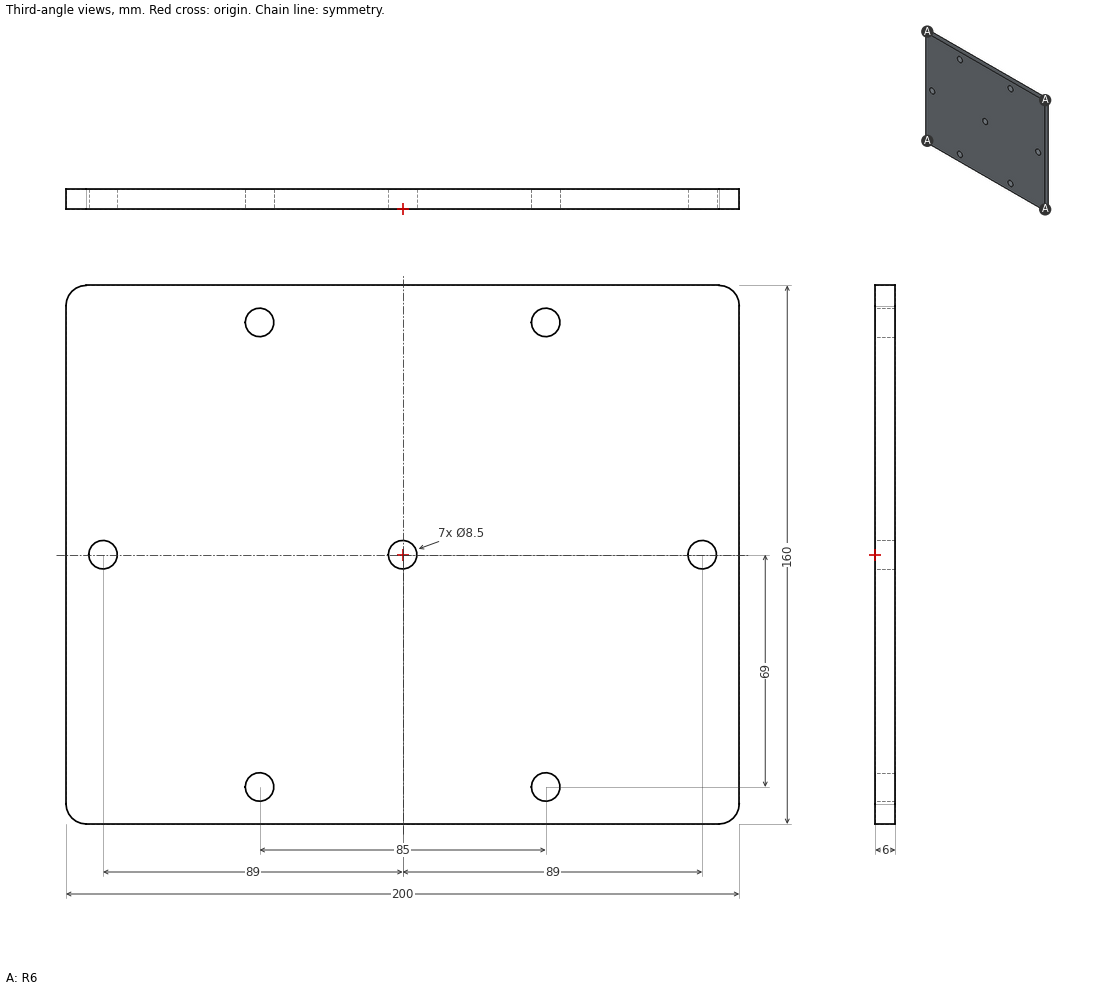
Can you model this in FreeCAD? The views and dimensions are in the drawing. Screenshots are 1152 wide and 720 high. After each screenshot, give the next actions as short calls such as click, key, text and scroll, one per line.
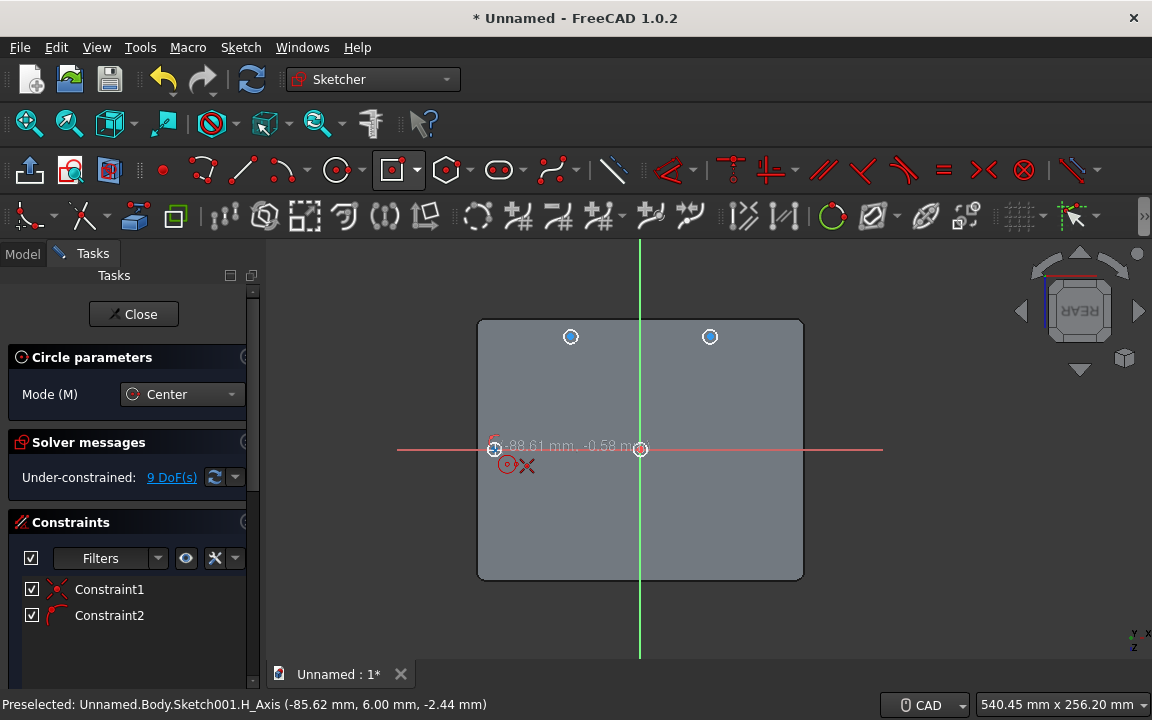
scroll(786, 450, up, 6)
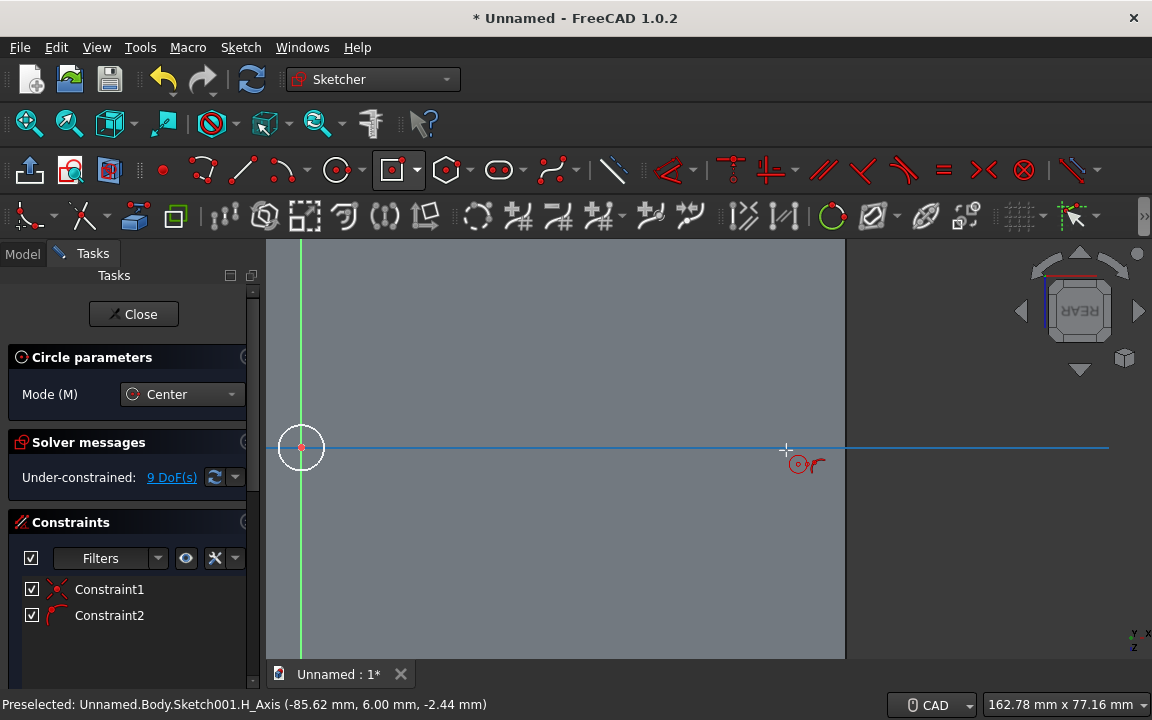
click(786, 448)
click(802, 431)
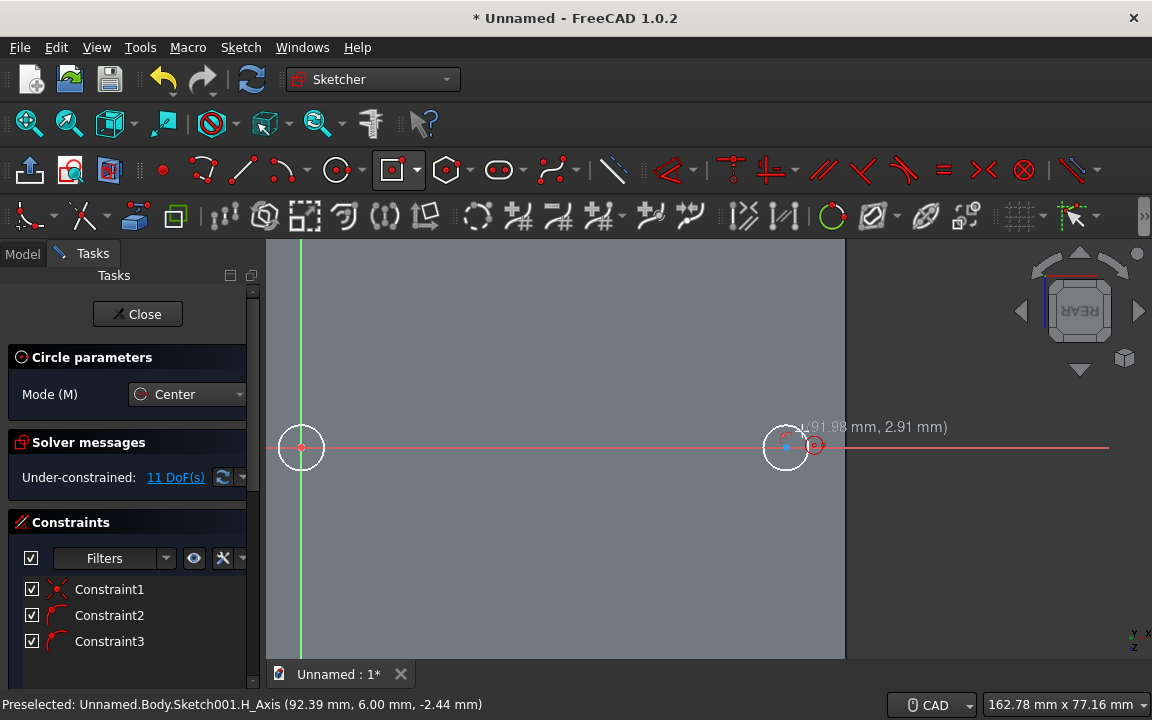
scroll(787, 450, down, 6)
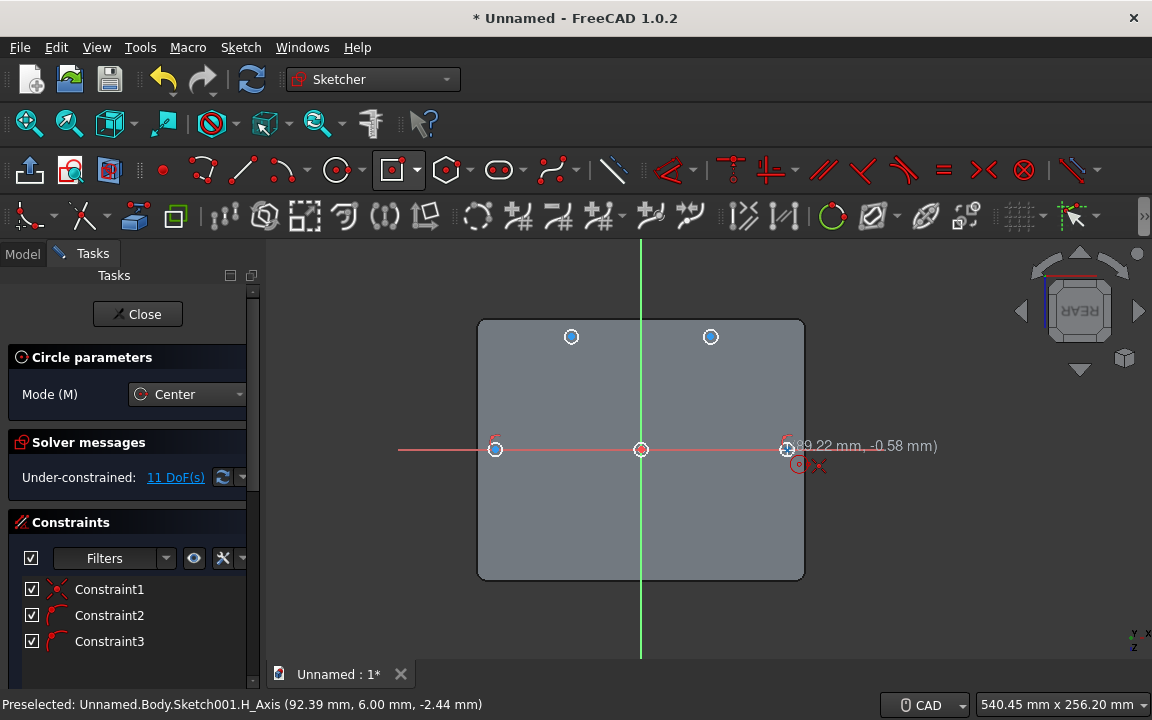
scroll(711, 563, up, 6)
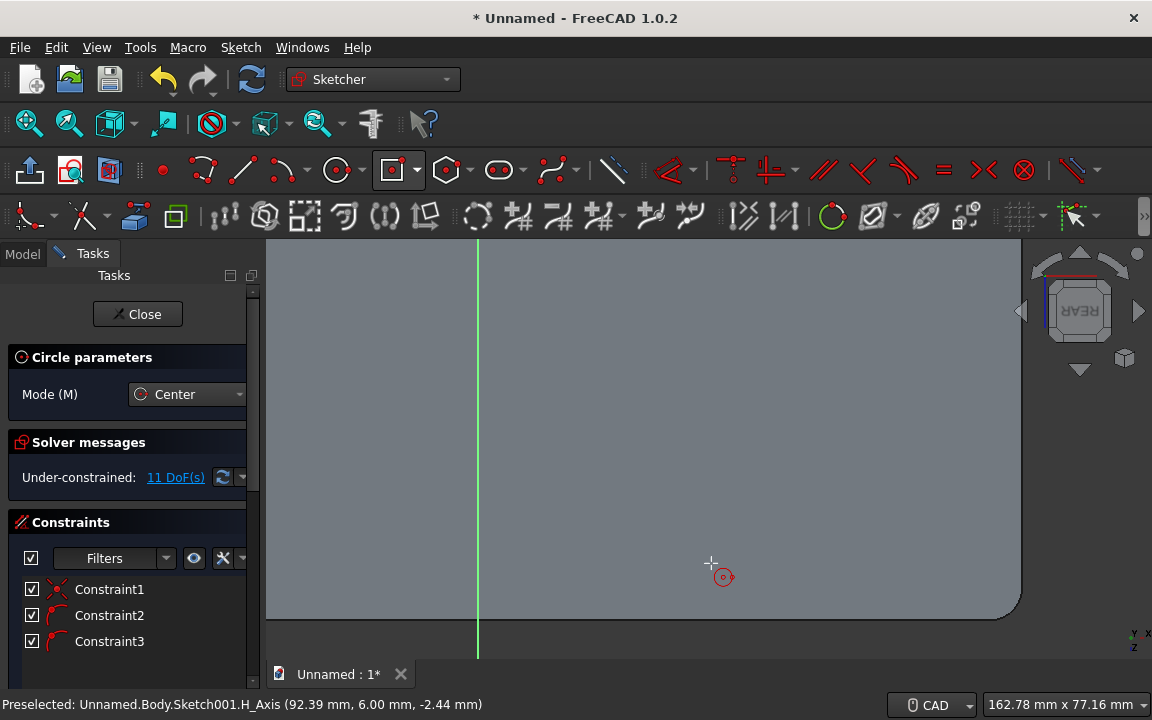
click(709, 561)
click(726, 544)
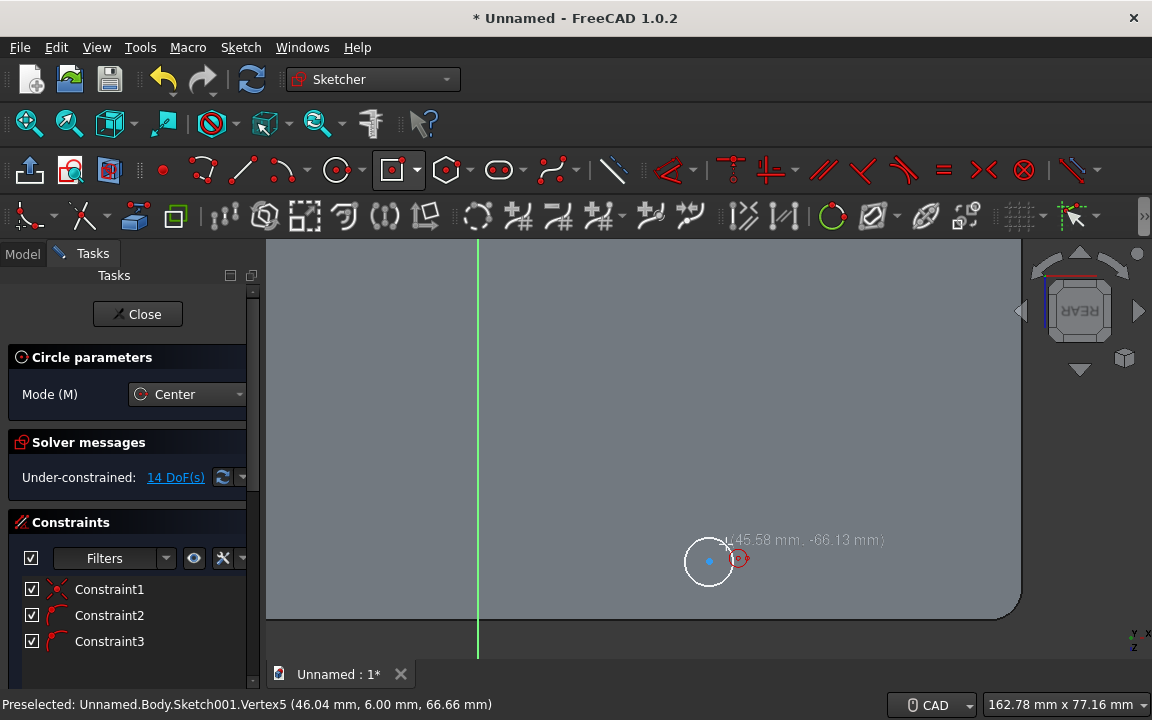
scroll(711, 563, down, 6)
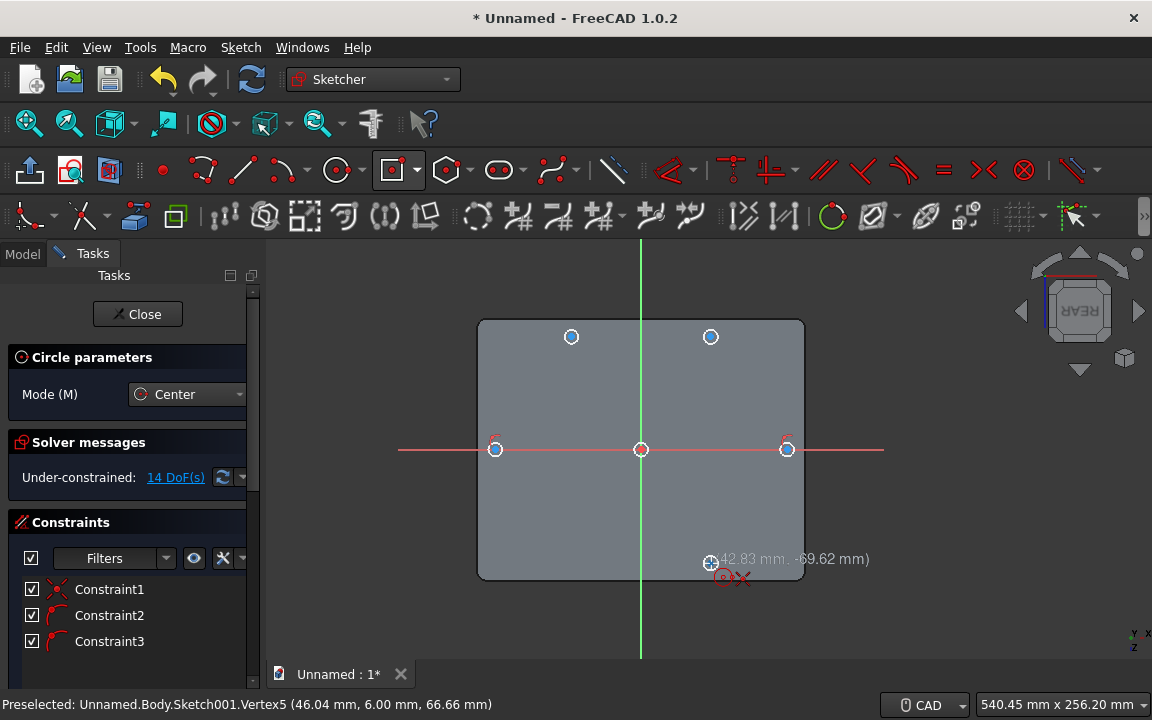
scroll(571, 563, up, 6)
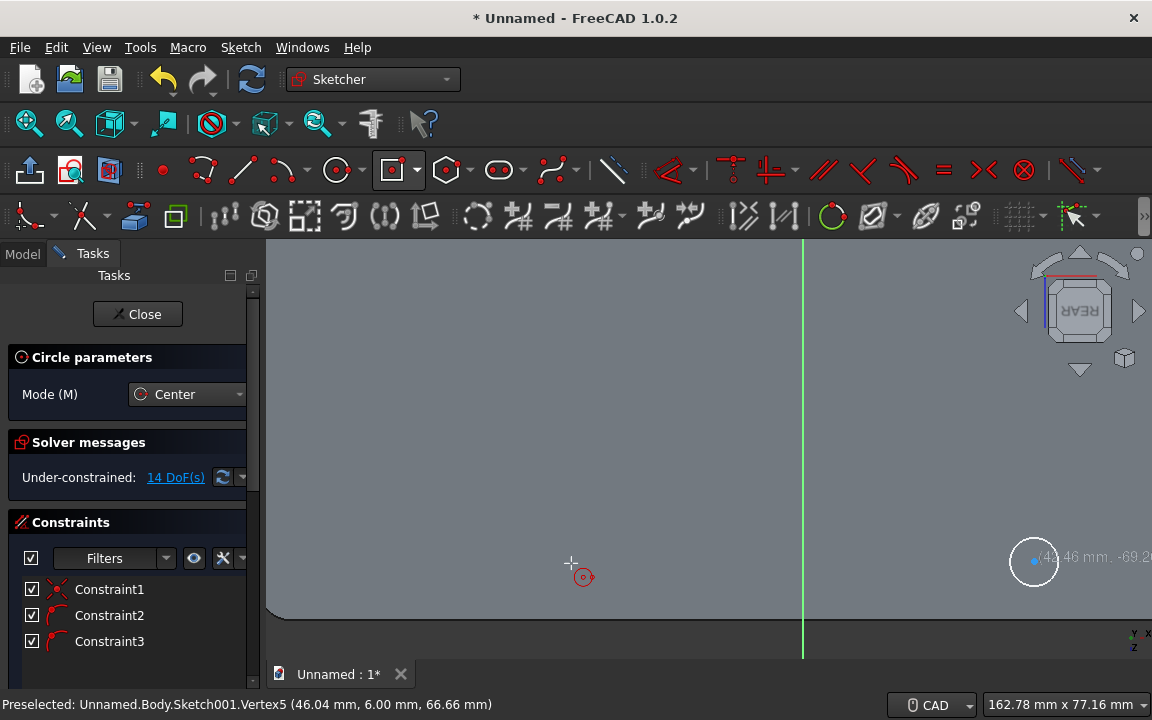
click(572, 561)
click(588, 544)
key(Escape)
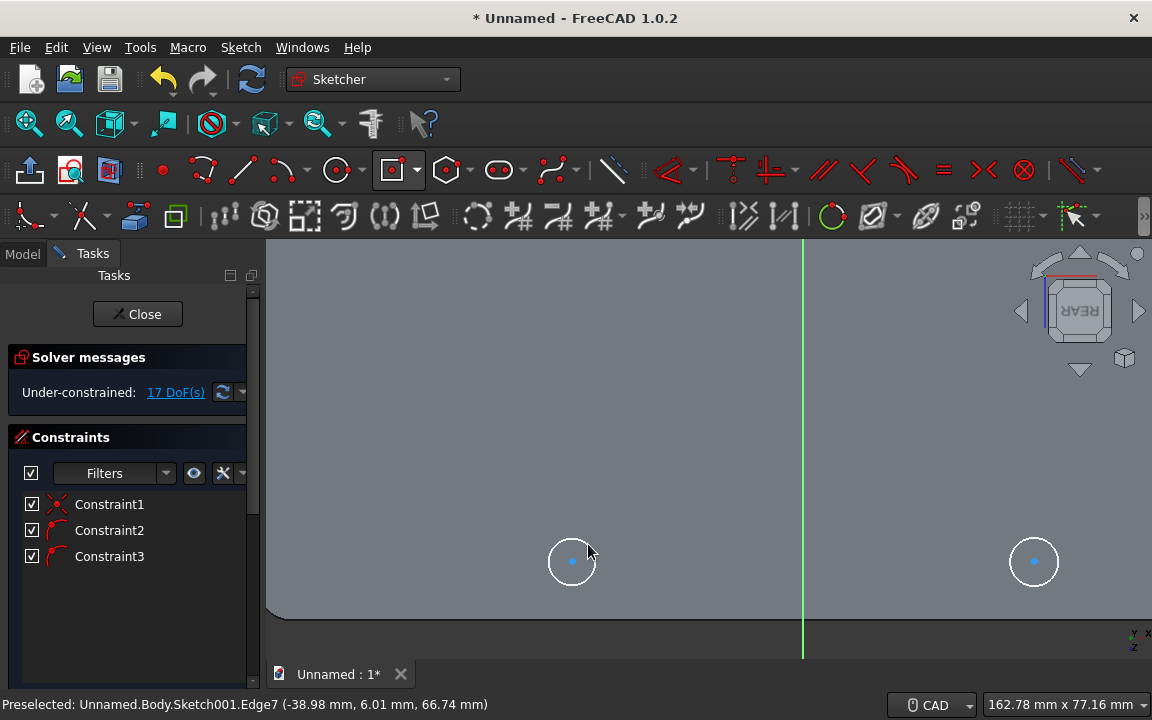
scroll(570, 563, down, 6)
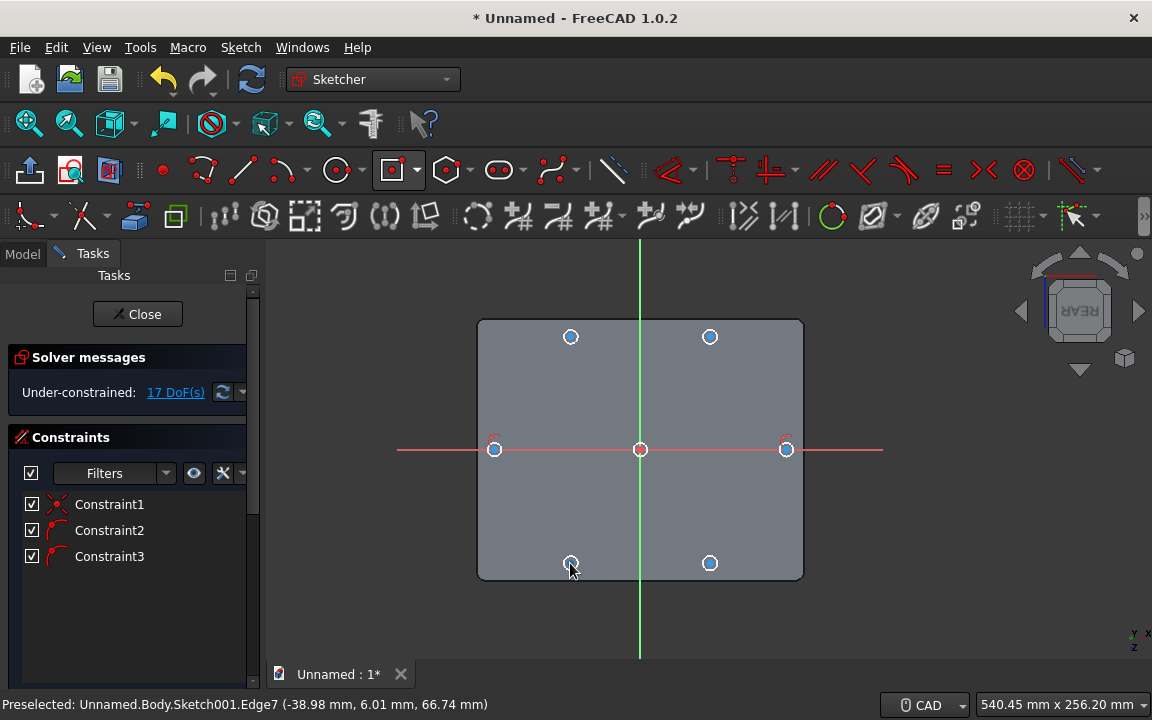
scroll(645, 445, up, 6)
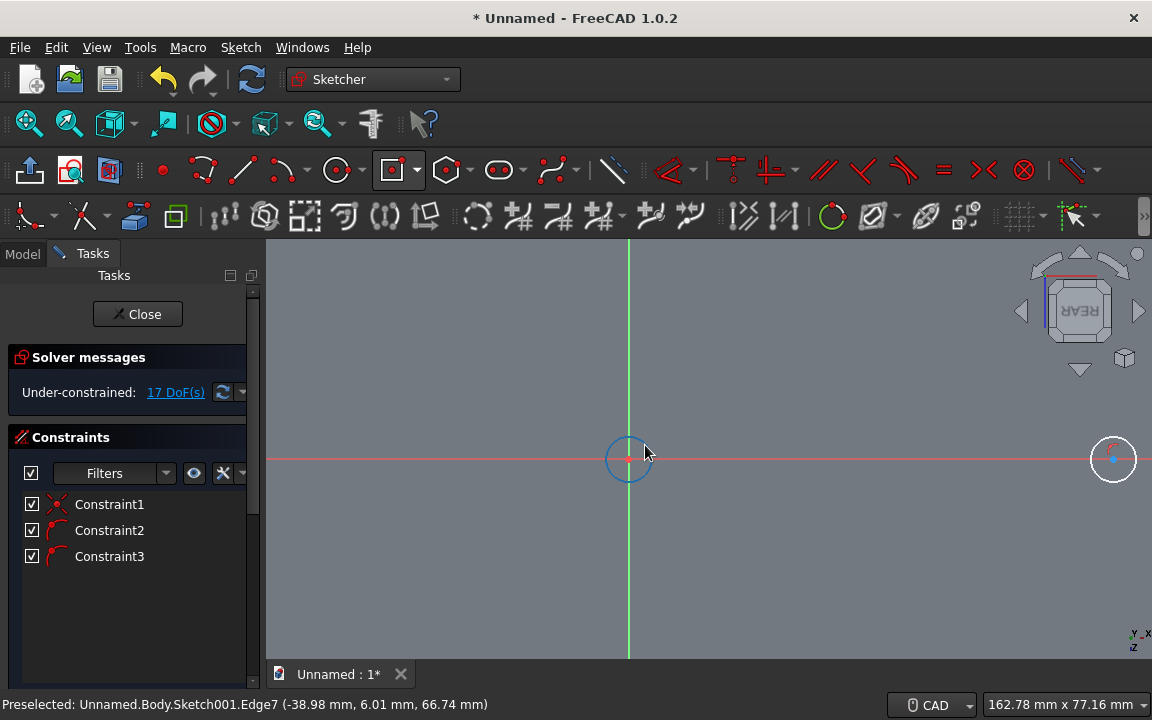
click(645, 443)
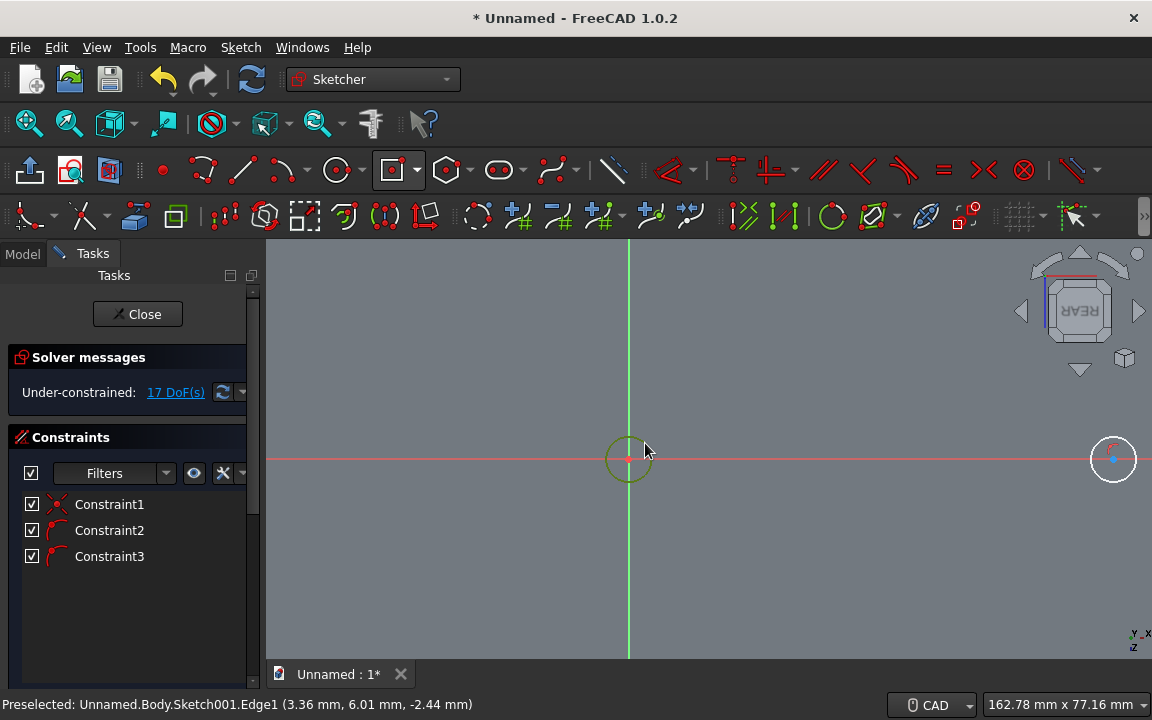
scroll(646, 444, down, 6)